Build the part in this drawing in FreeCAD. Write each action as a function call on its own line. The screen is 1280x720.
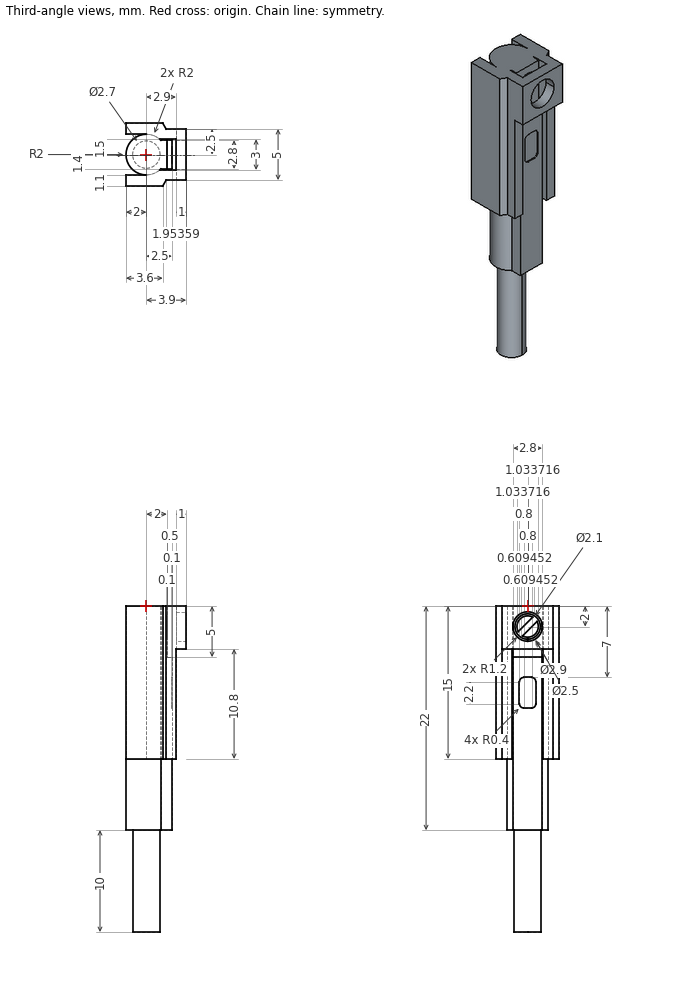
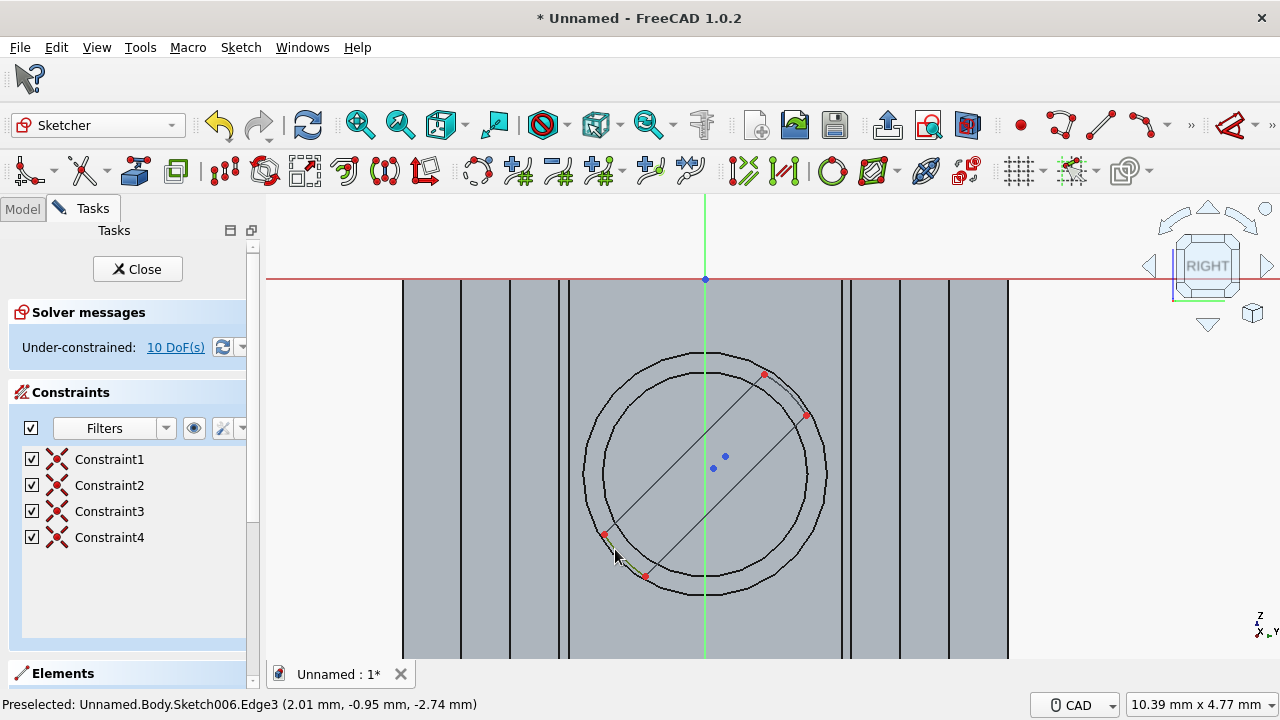
click(796, 401)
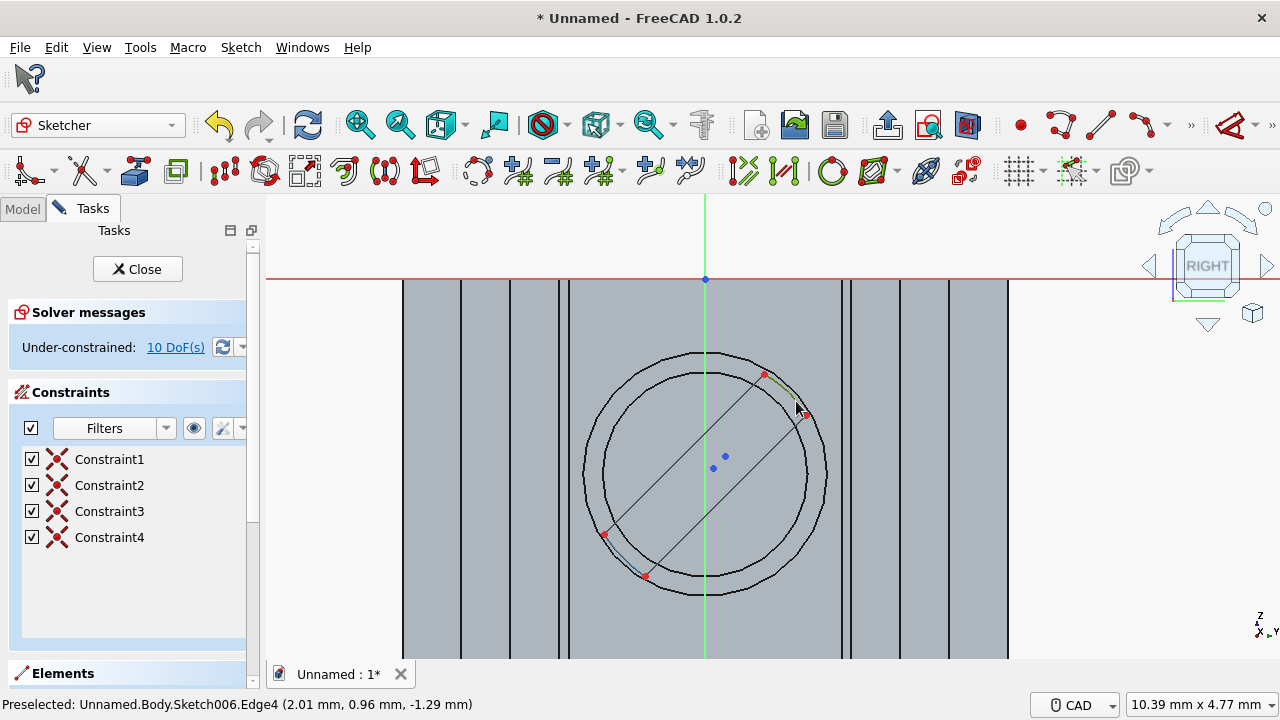
key(c)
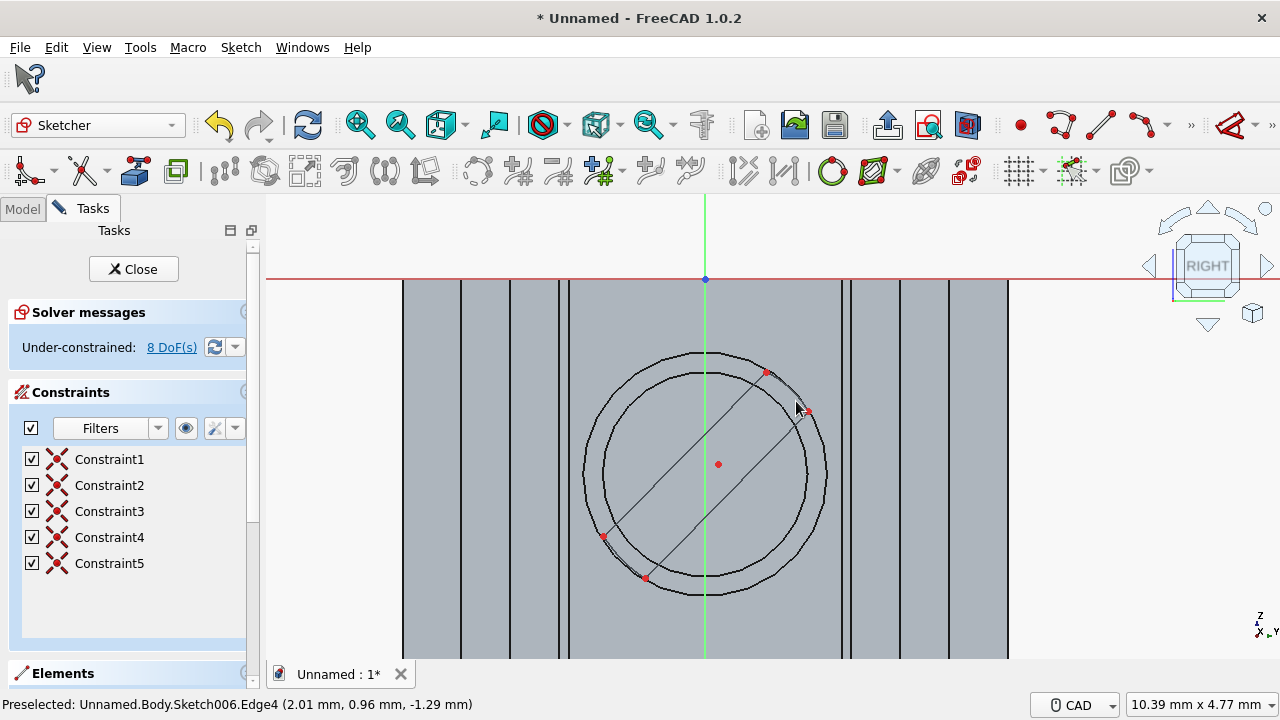
click(614, 551)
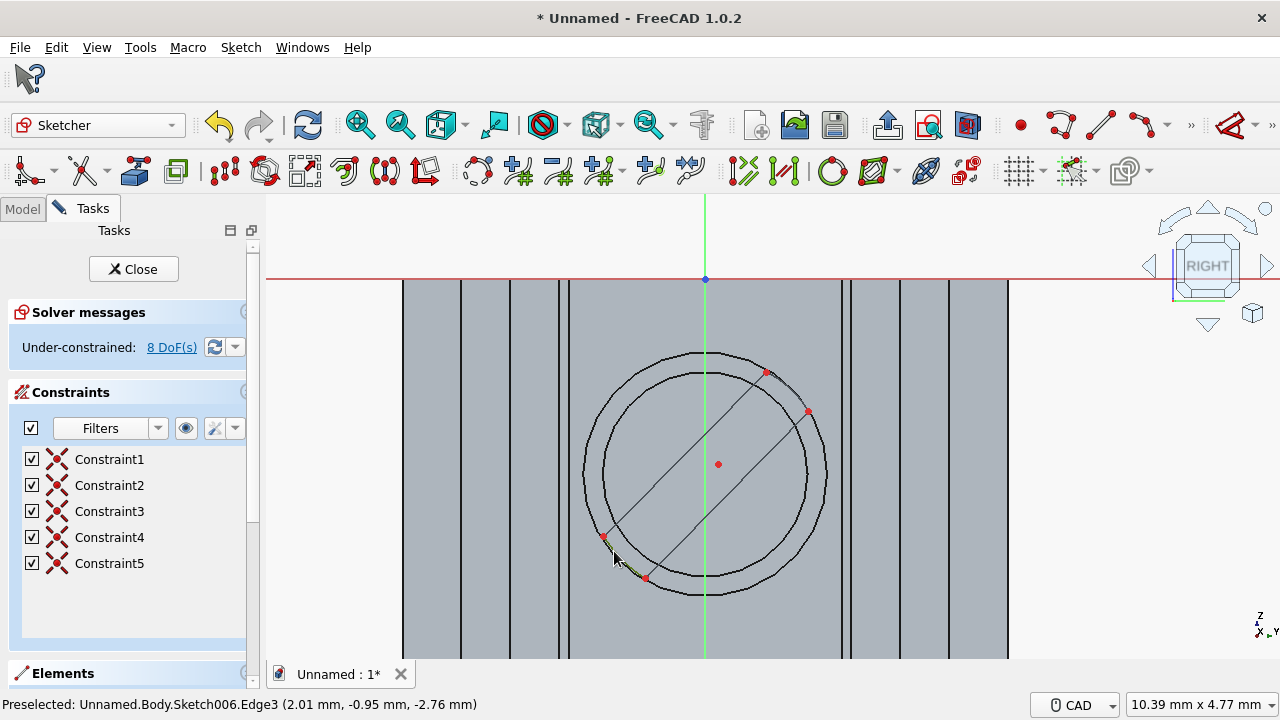
click(799, 397)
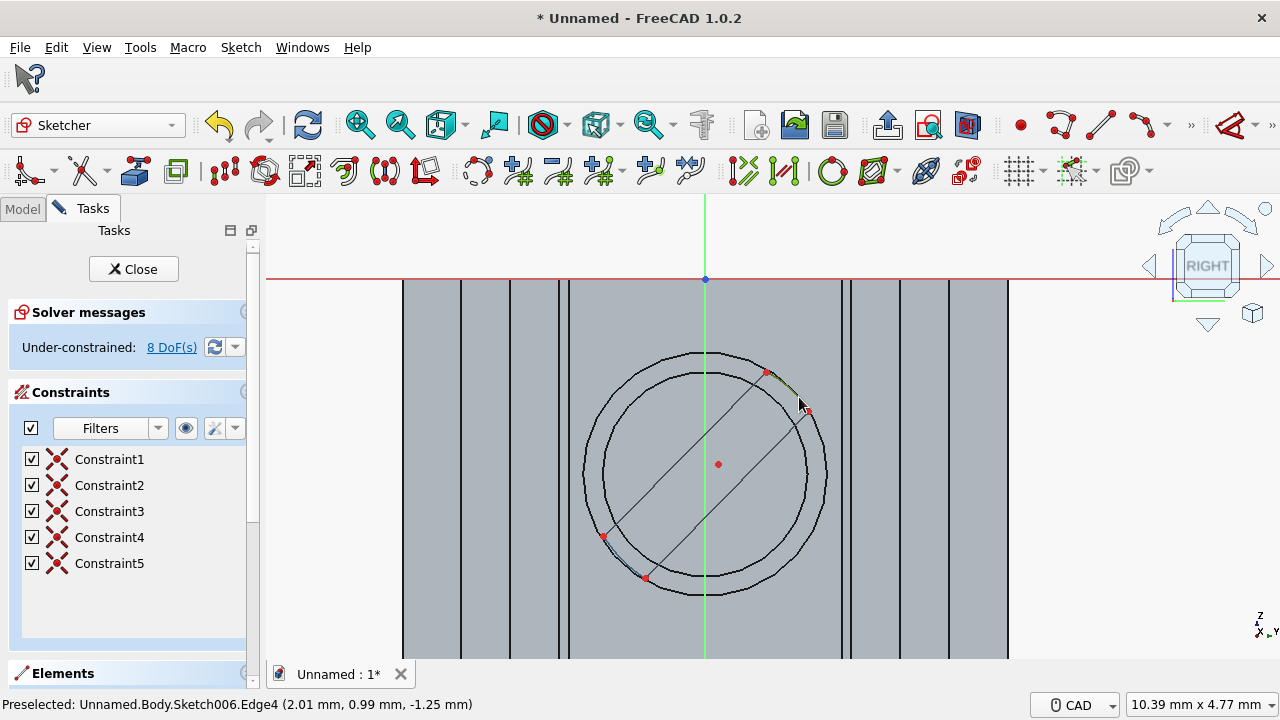
key(e)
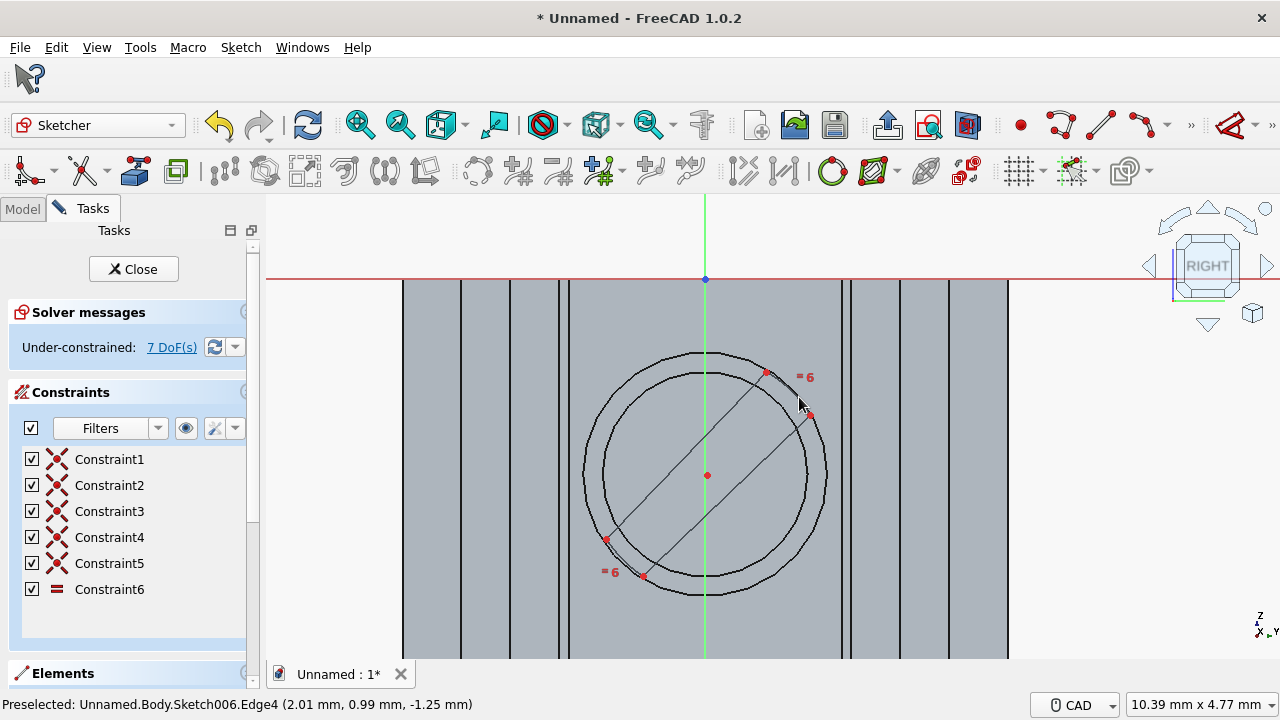
click(708, 476)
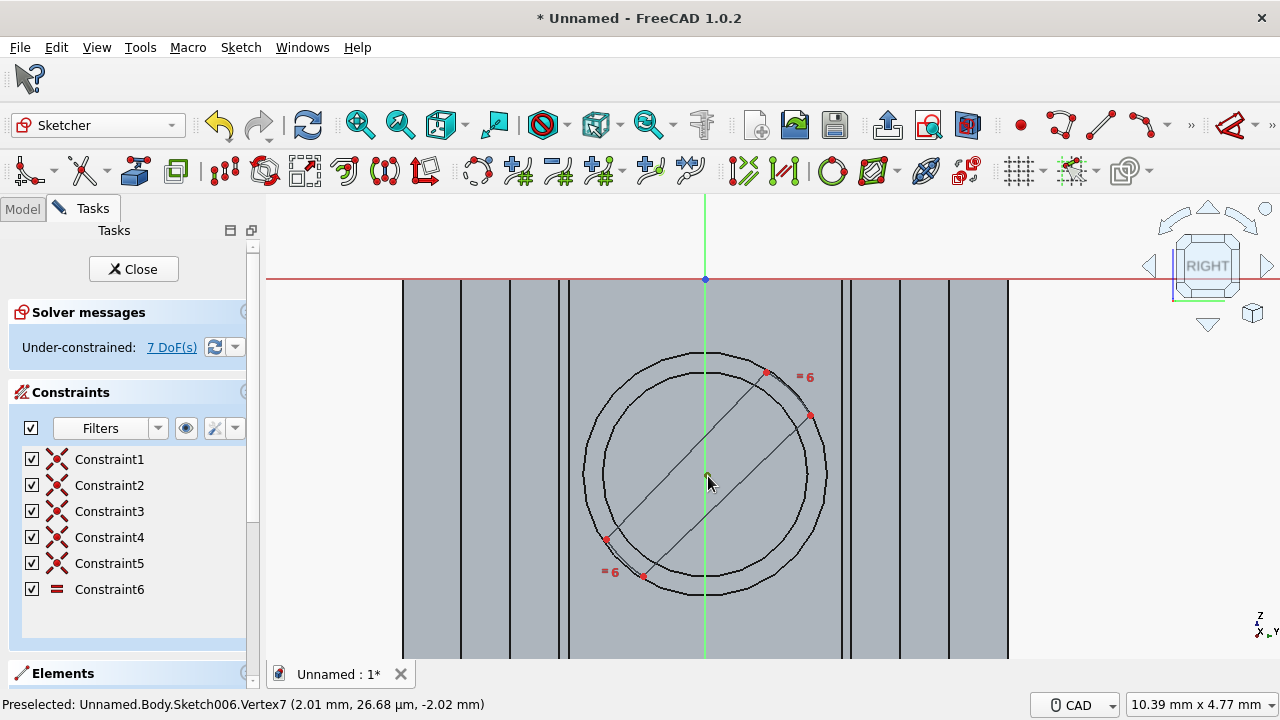
click(705, 602)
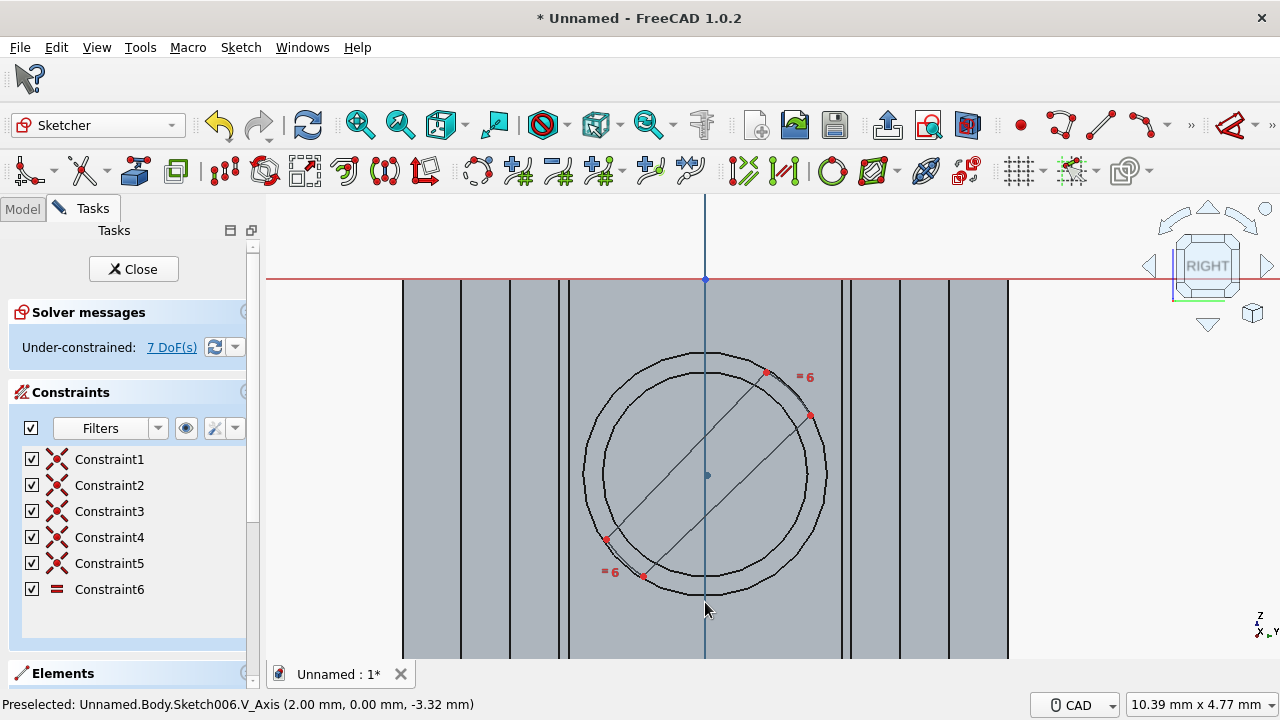
key(c)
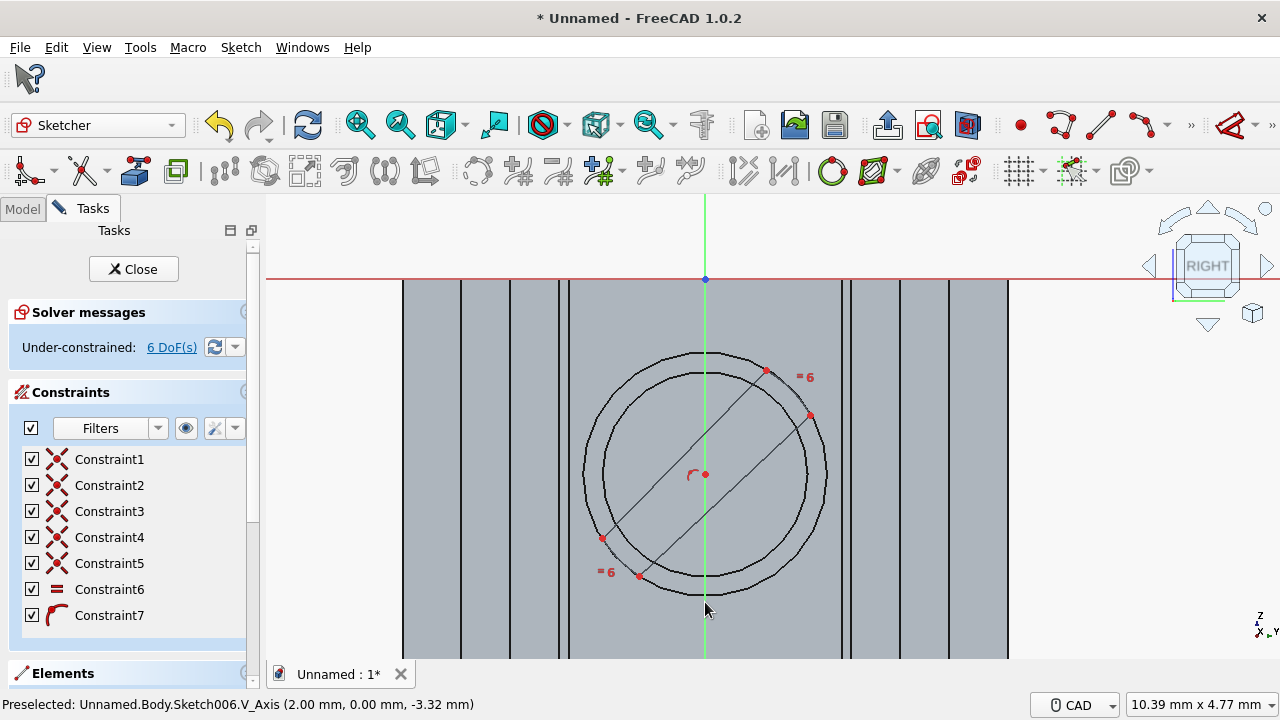
click(1230, 126)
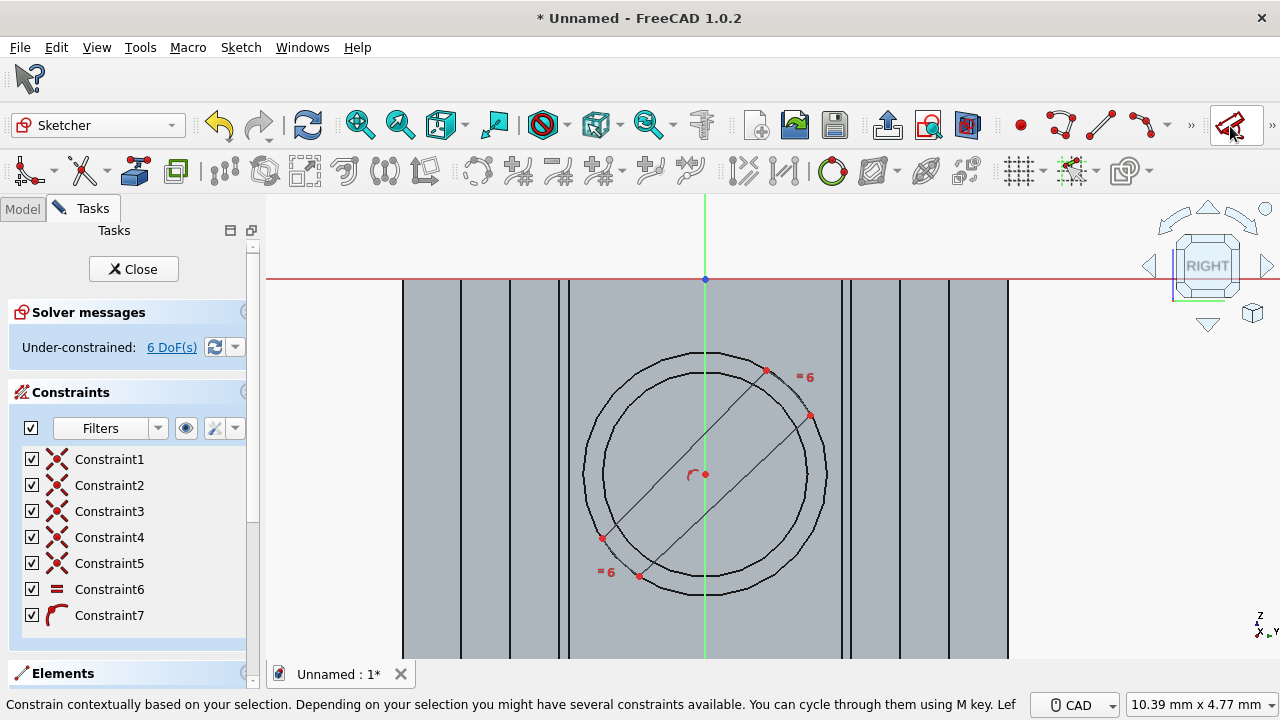
click(612, 552)
click(587, 572)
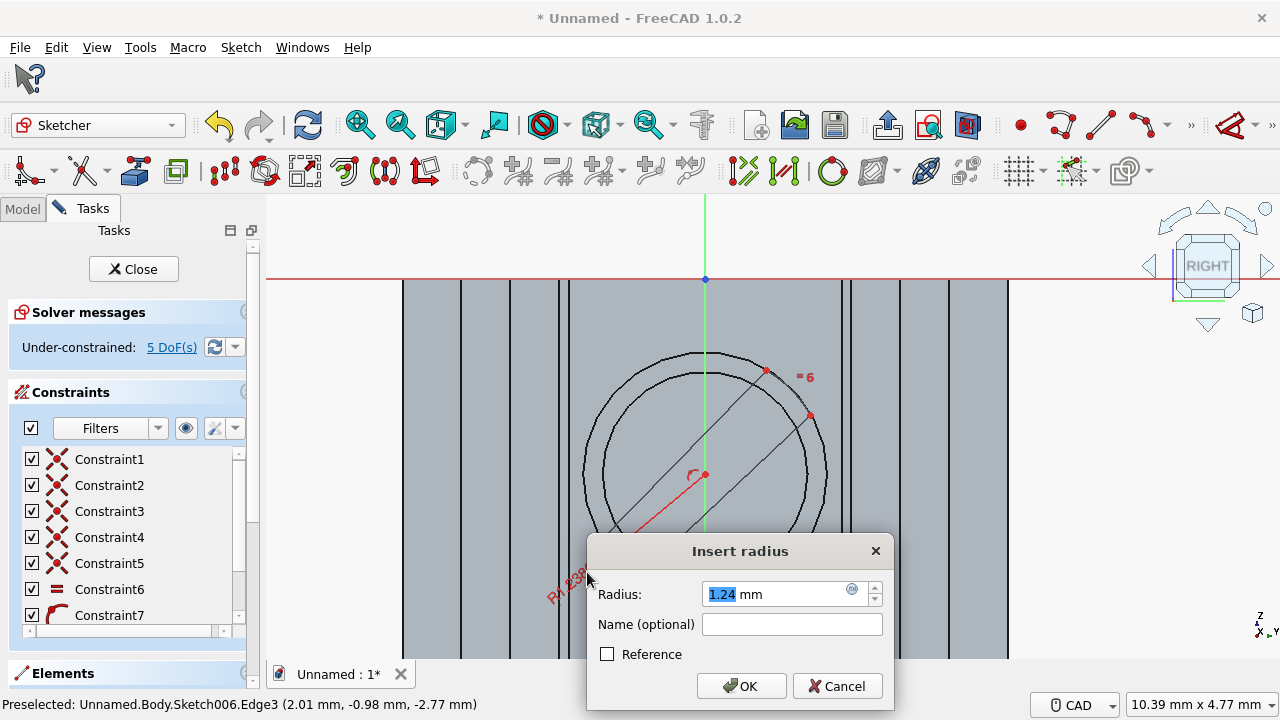
text(1.2)
key(Return)